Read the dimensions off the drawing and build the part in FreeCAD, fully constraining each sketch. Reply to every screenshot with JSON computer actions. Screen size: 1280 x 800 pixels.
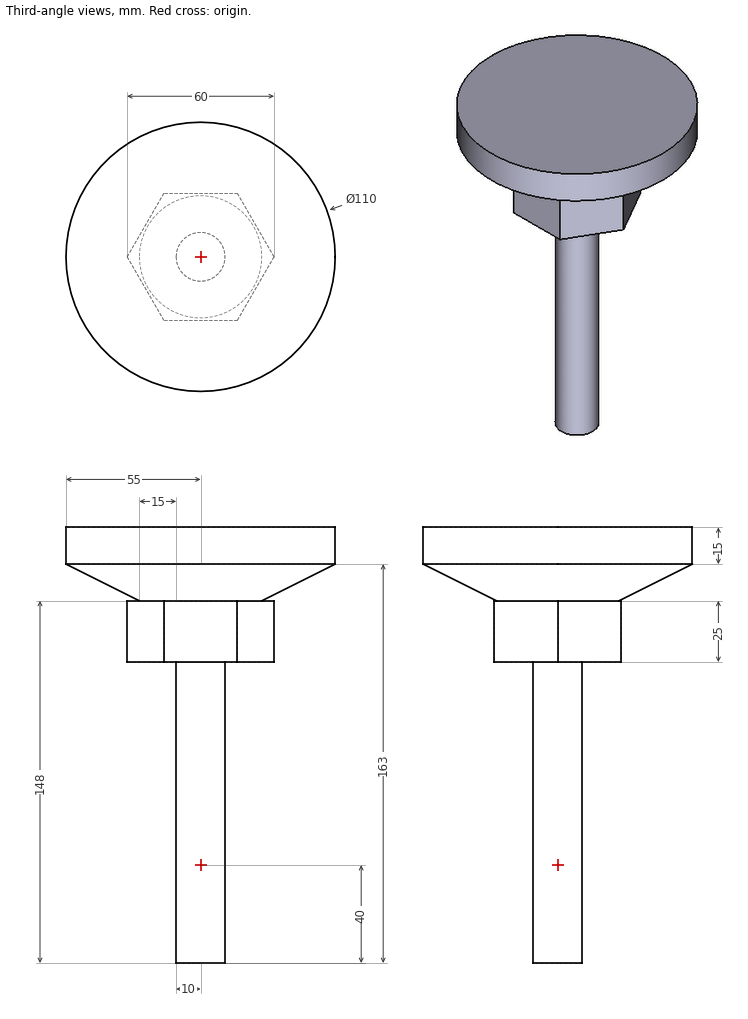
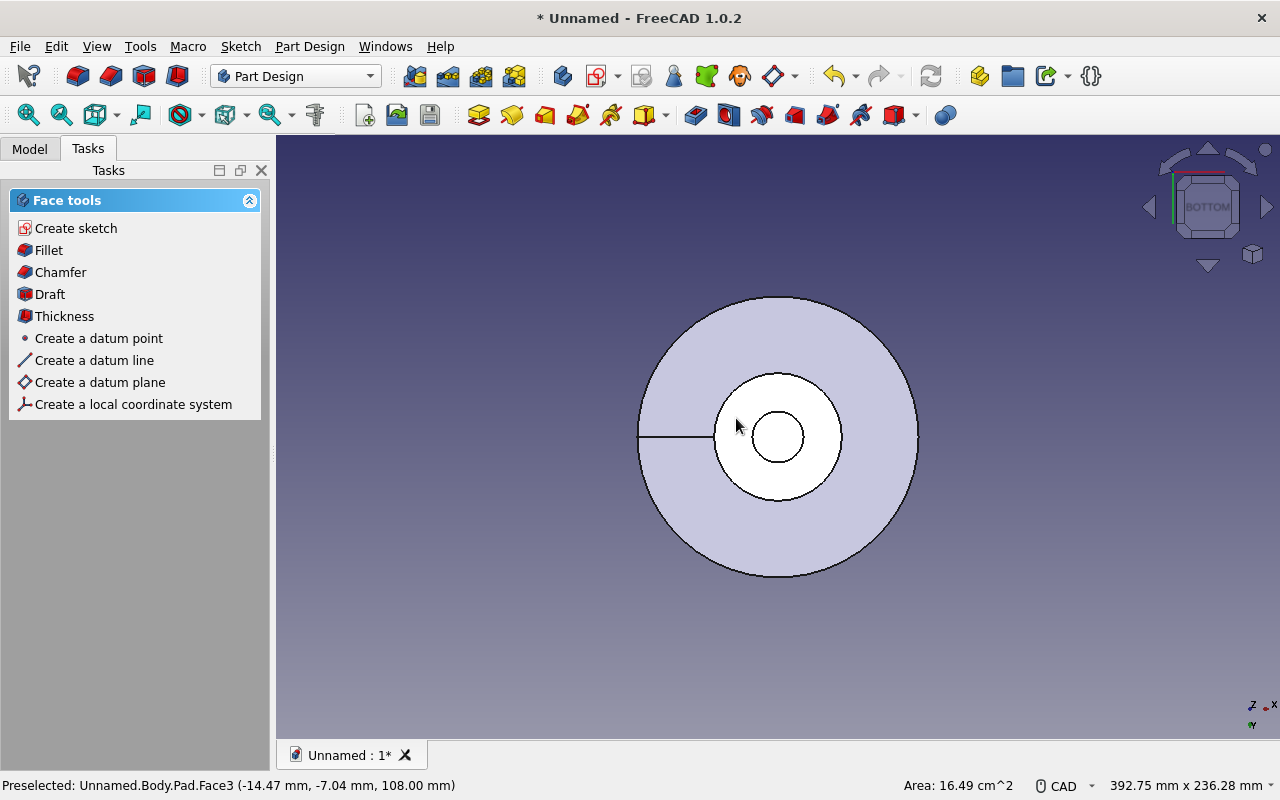
{"action": "left_click", "coordinate": [596, 76]}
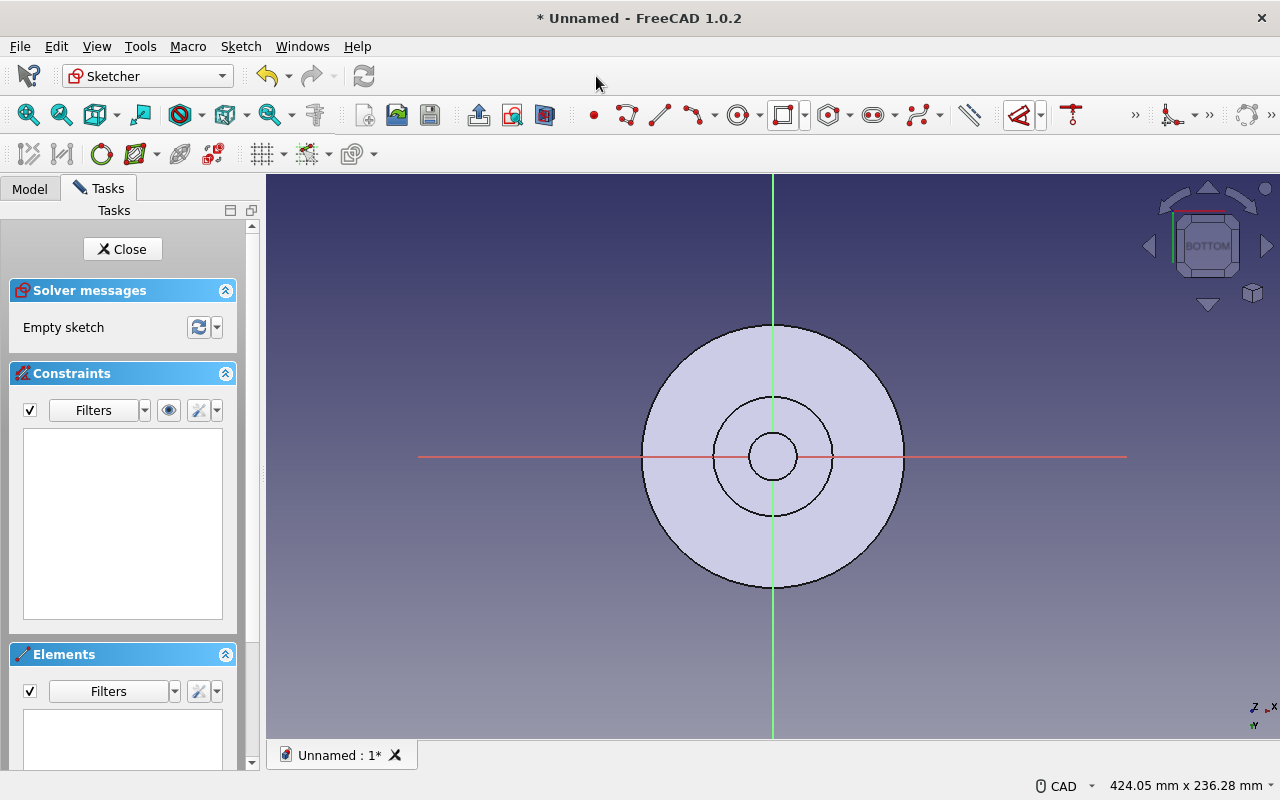
{"action": "scroll", "coordinate": [813, 457], "scroll_direction": "up", "scroll_amount": 5}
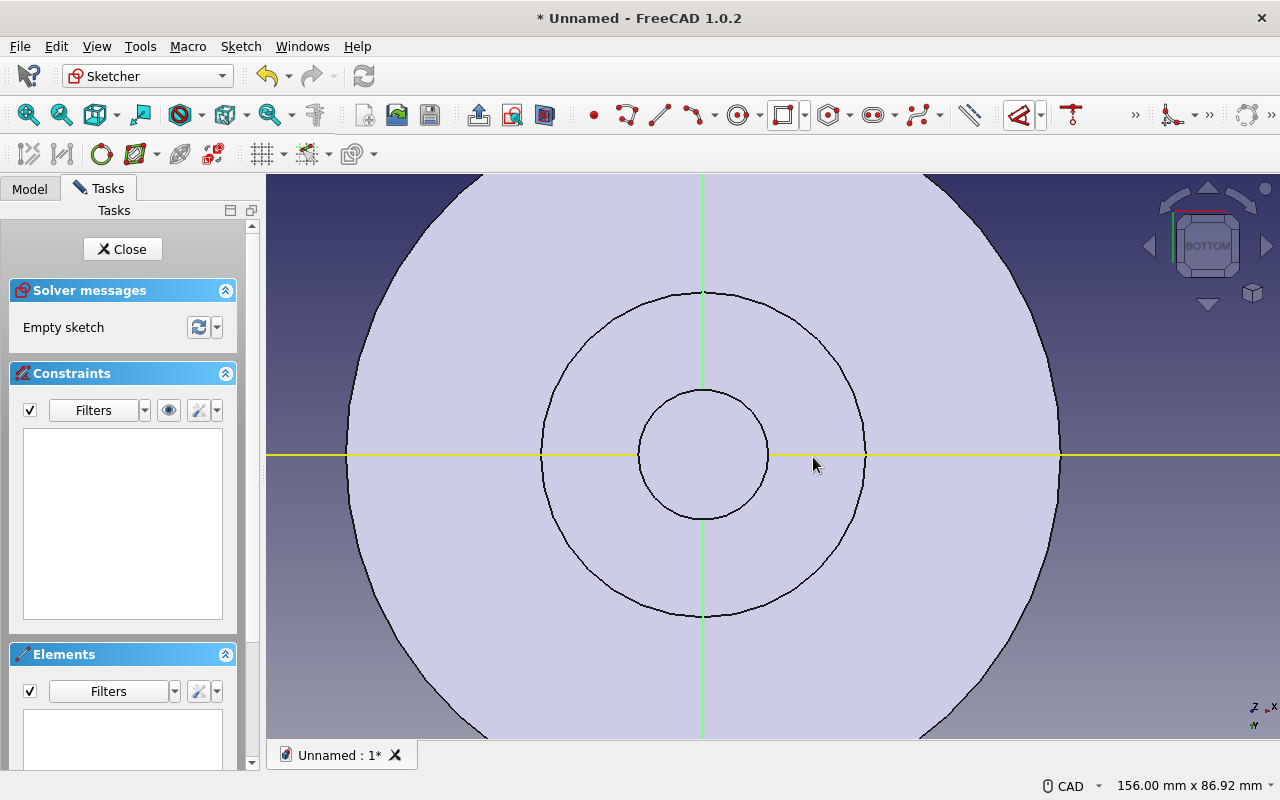
{"action": "left_click", "coordinate": [828, 116]}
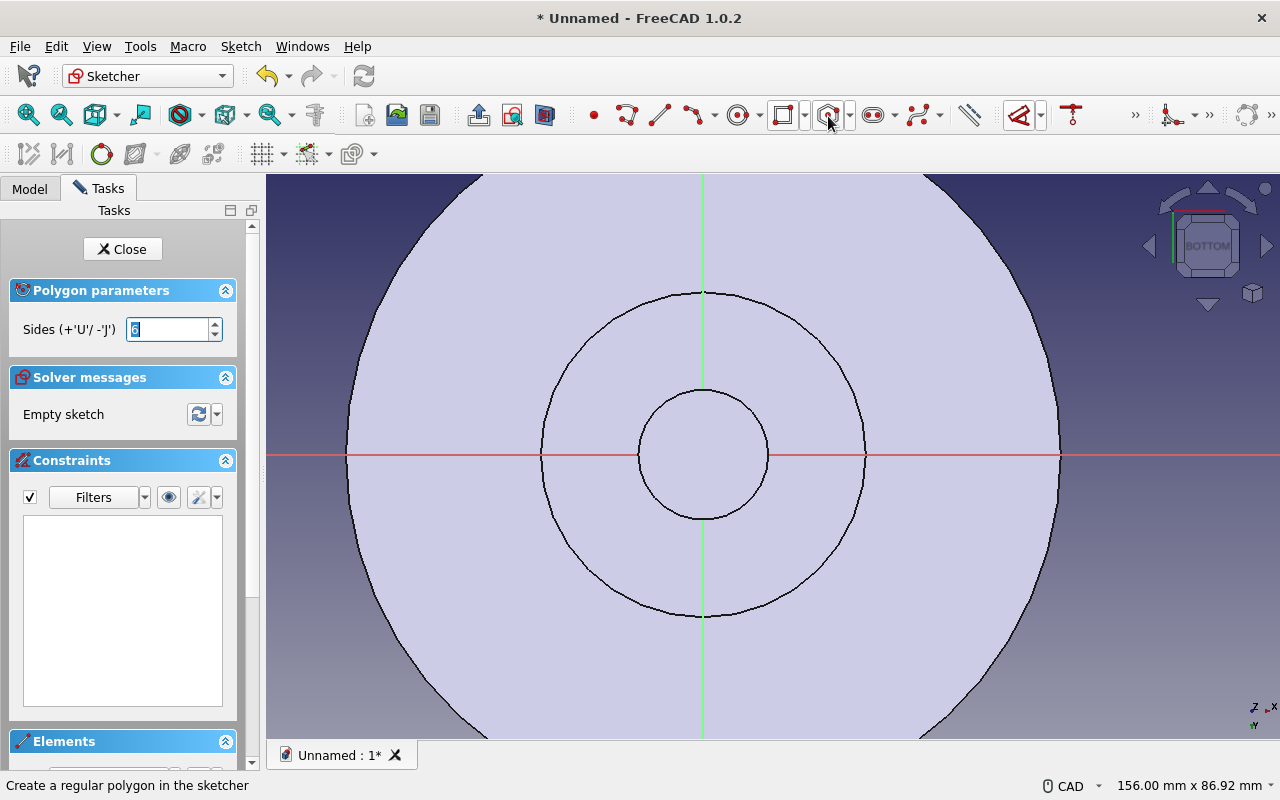
{"action": "left_click", "coordinate": [703, 455]}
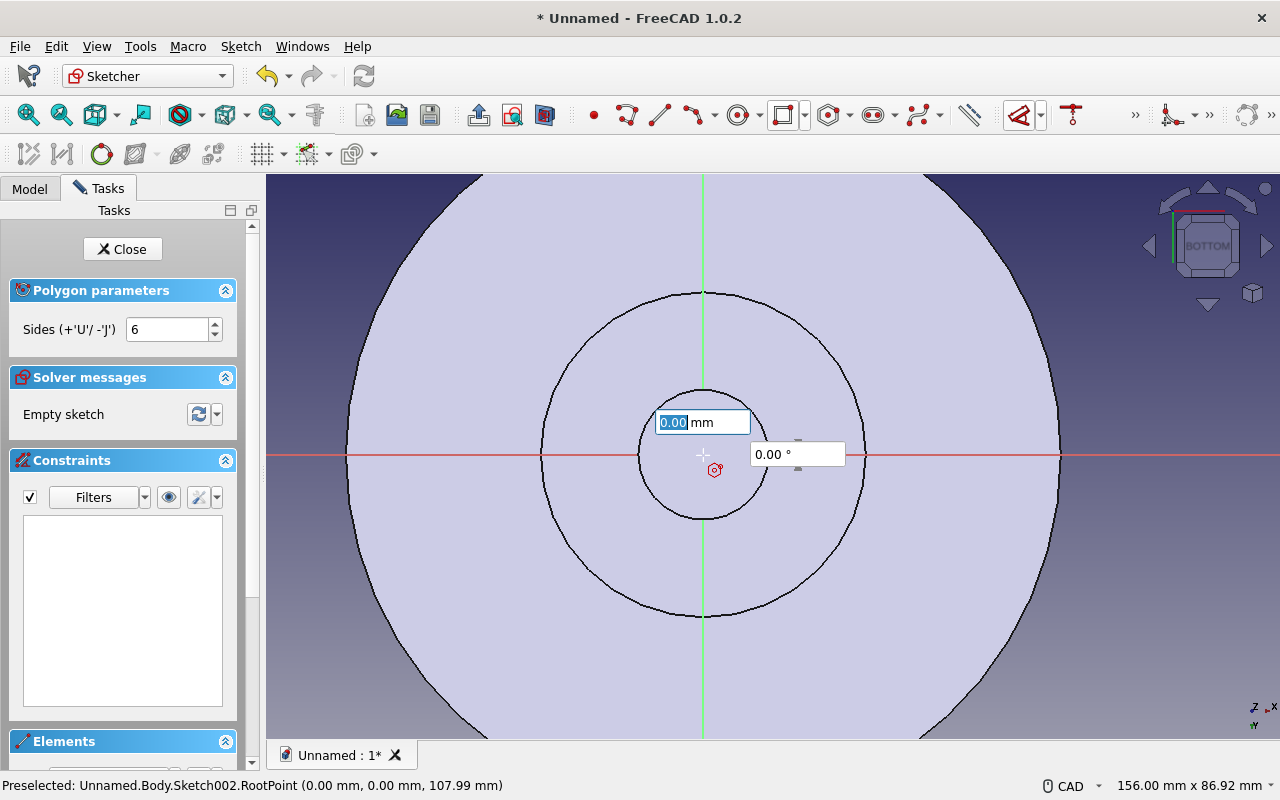
{"action": "left_click", "coordinate": [898, 455]}
{"action": "right_click", "coordinate": [898, 455]}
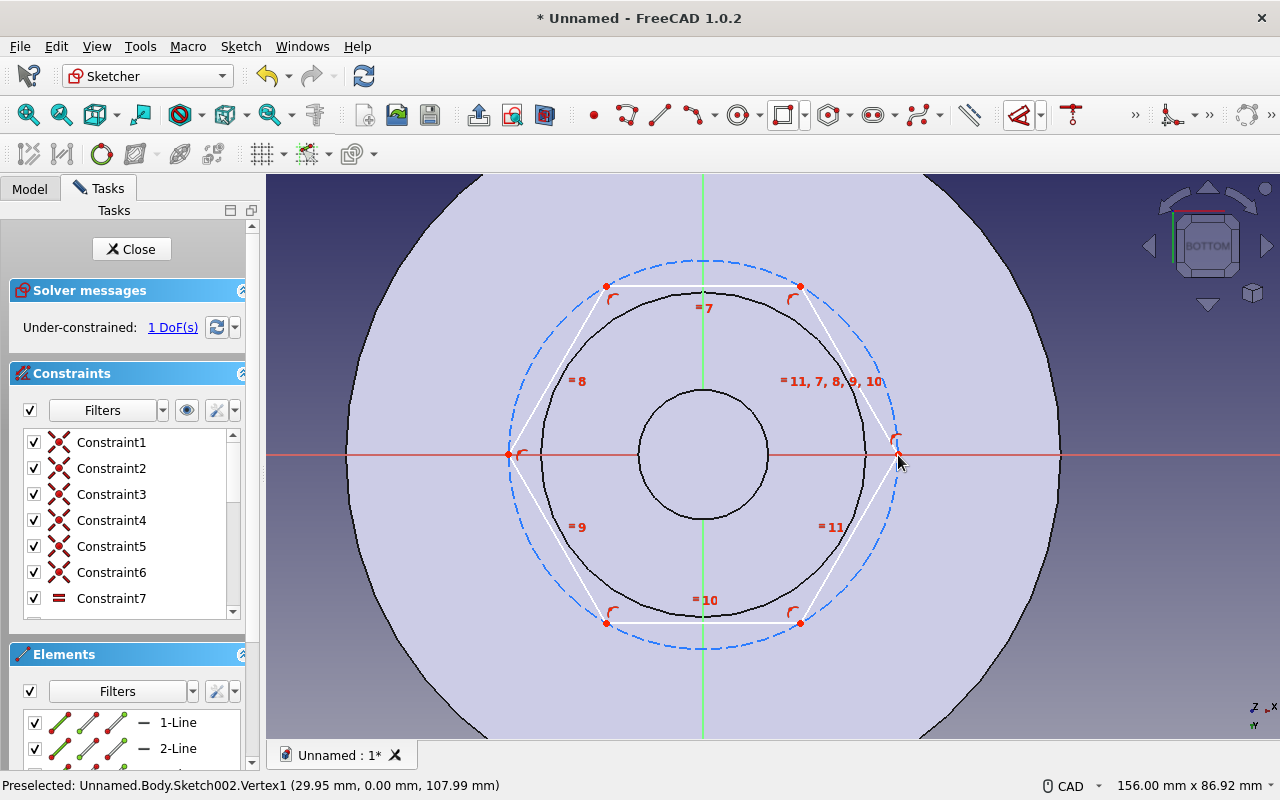
{"action": "left_click", "coordinate": [509, 455]}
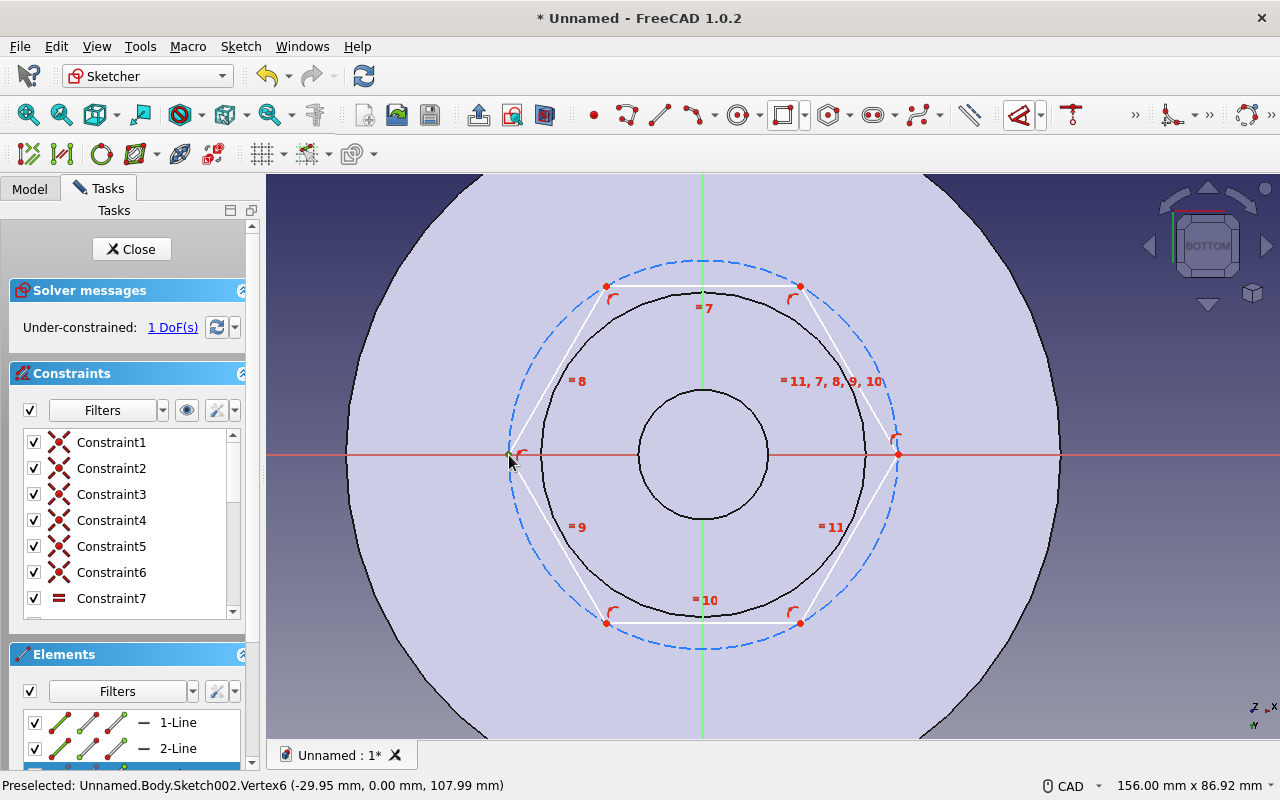
{"action": "left_click", "coordinate": [898, 455]}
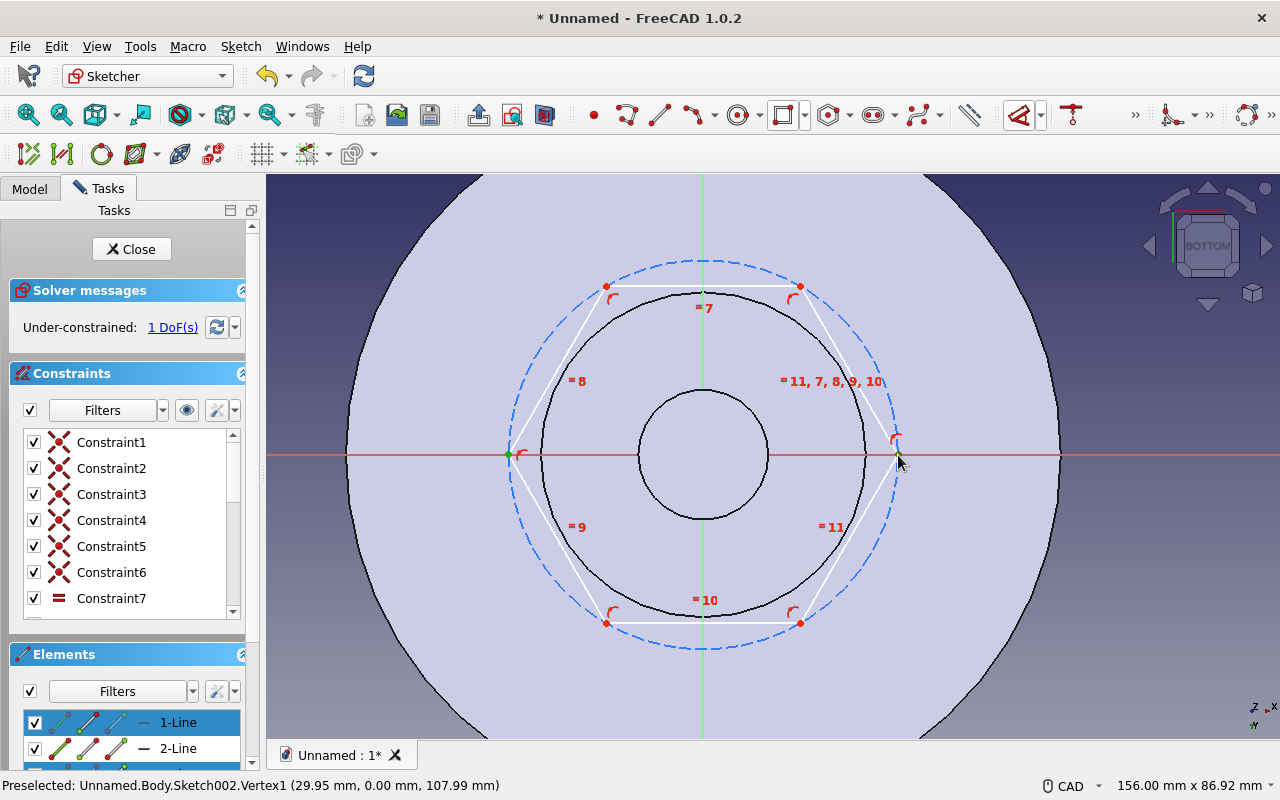
{"action": "key", "text": "l"}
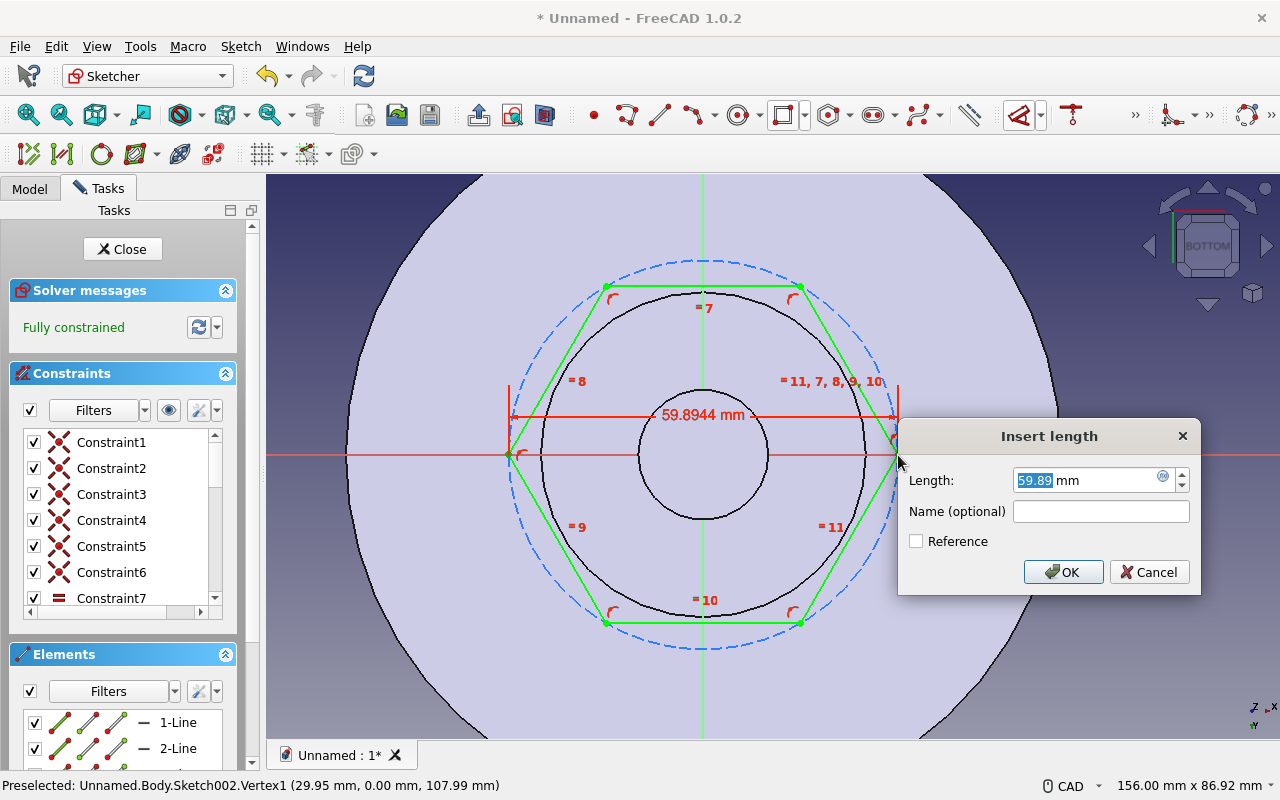
{"action": "type", "text": "60"}
{"action": "key", "text": "Return"}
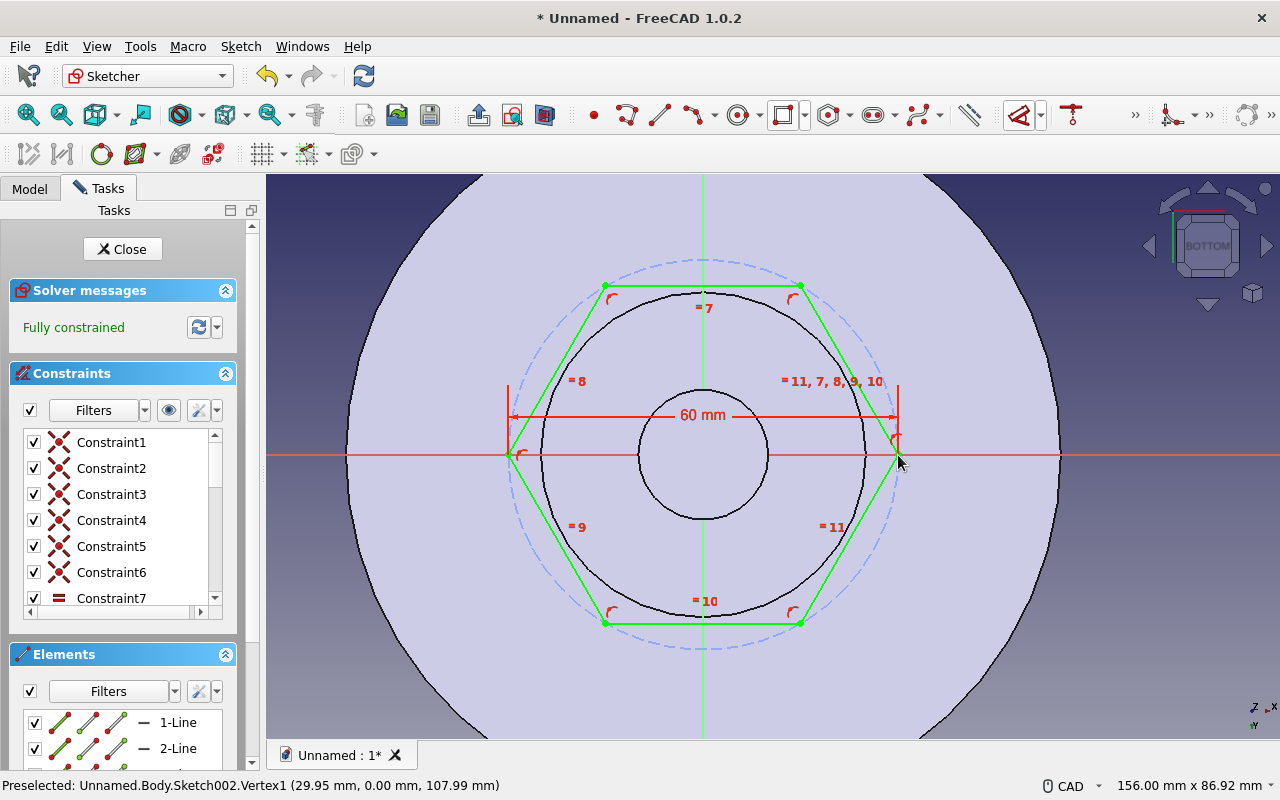
{"action": "left_click", "coordinate": [123, 249]}